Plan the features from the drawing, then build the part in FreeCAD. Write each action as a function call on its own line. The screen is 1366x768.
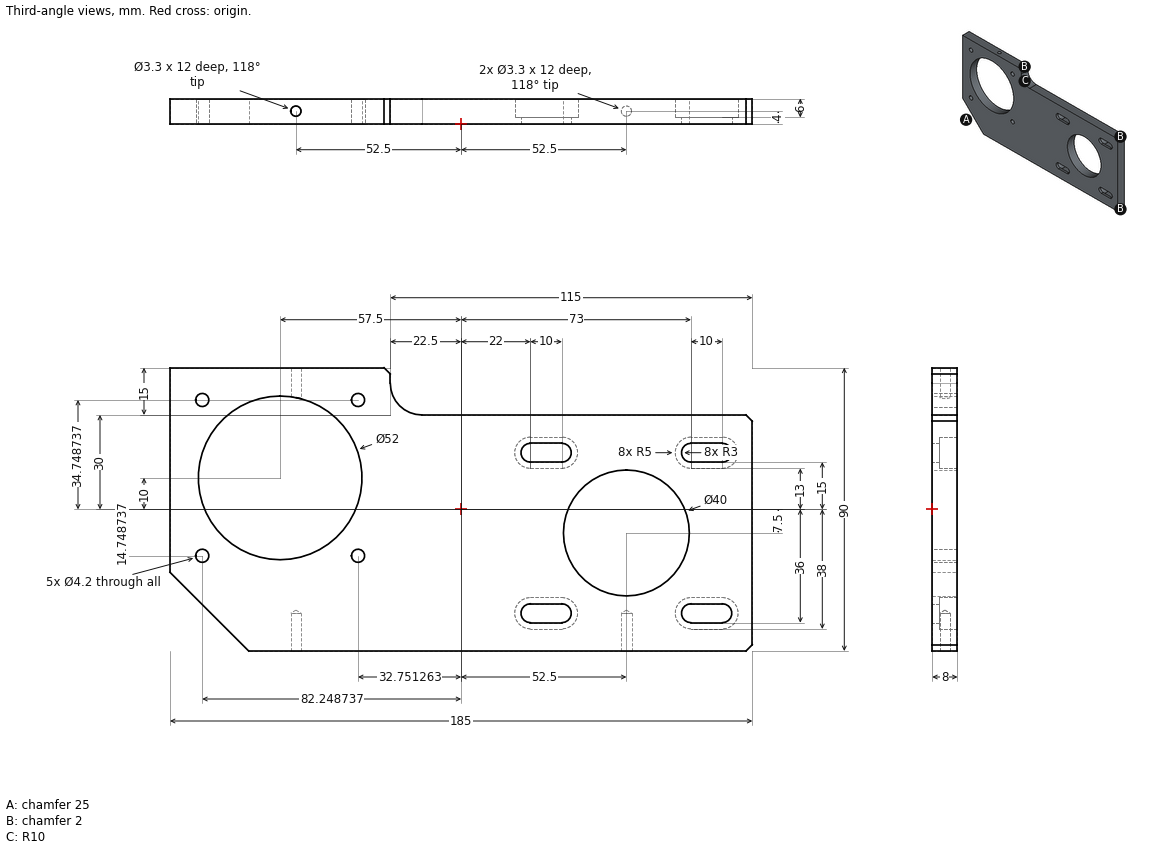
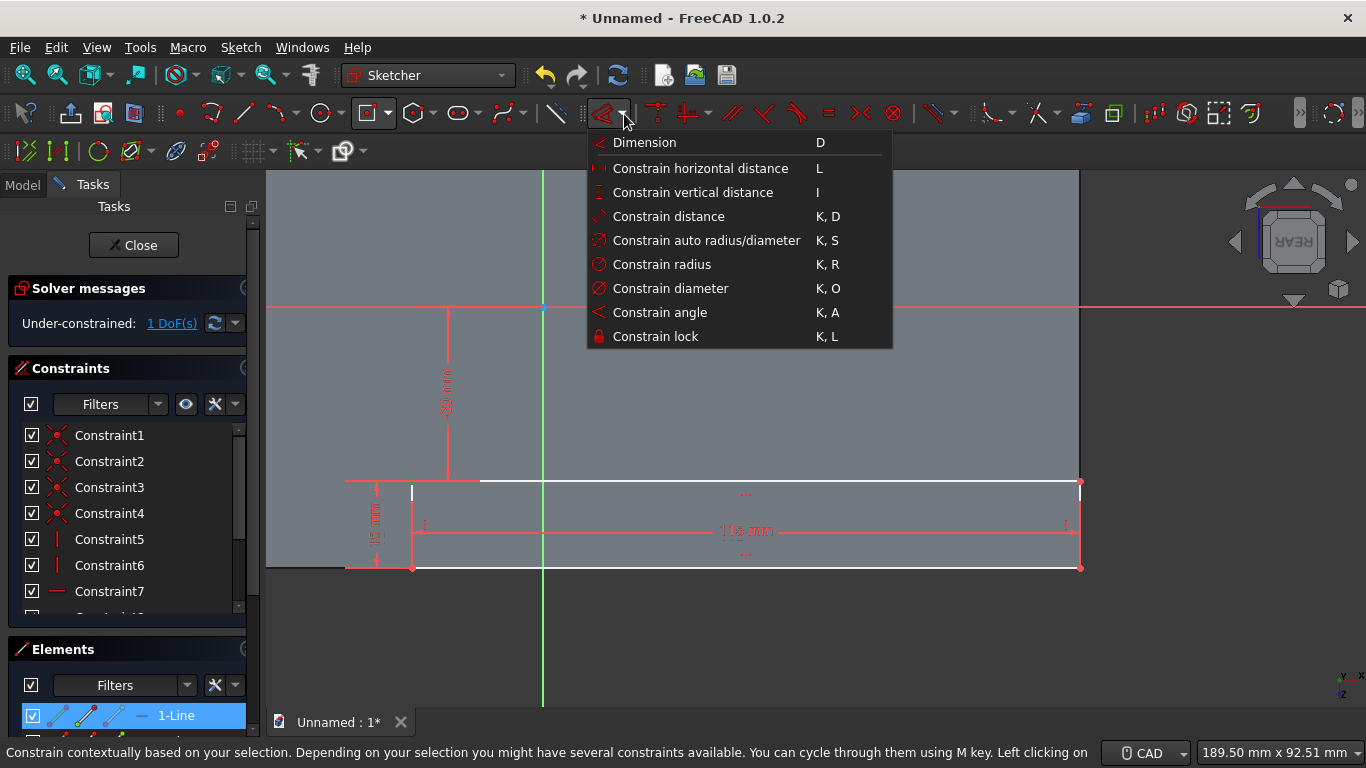
click(740, 168)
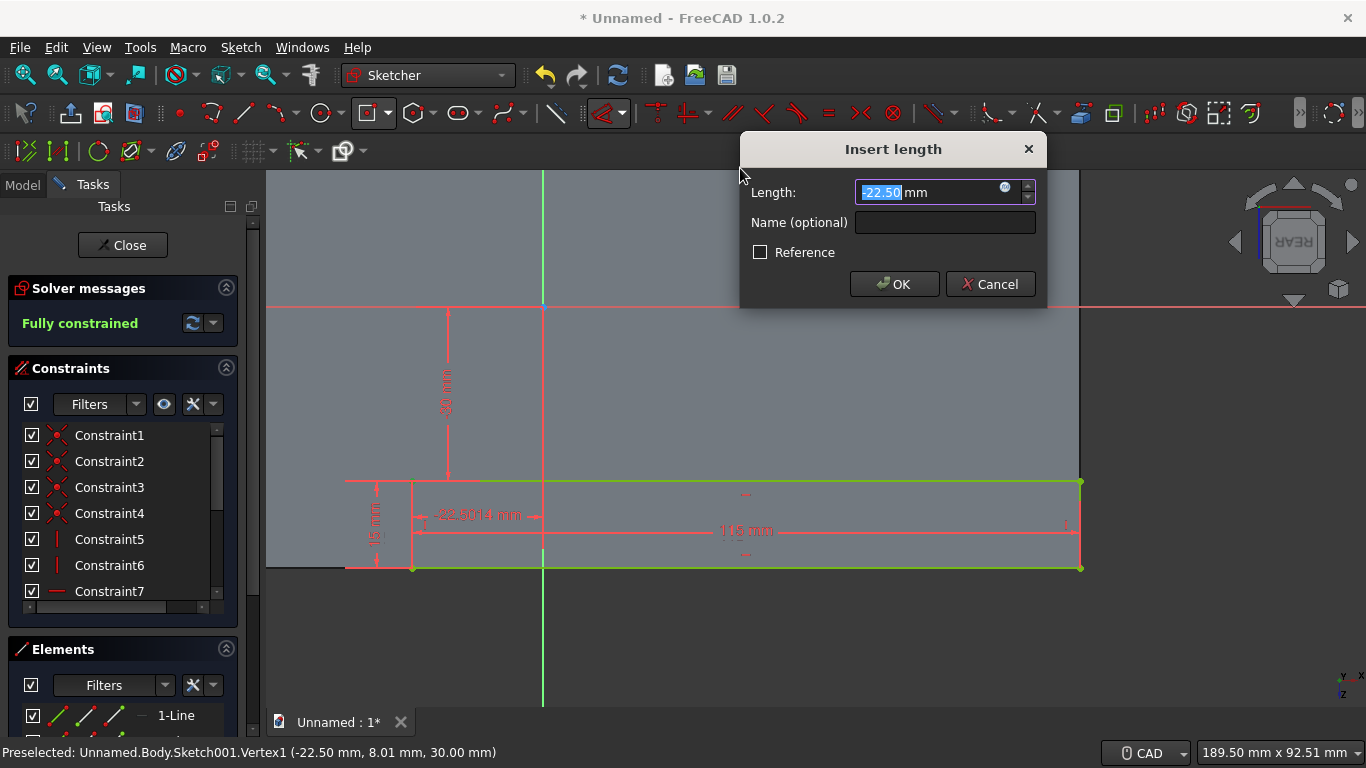
text(-22.5)
key(Return)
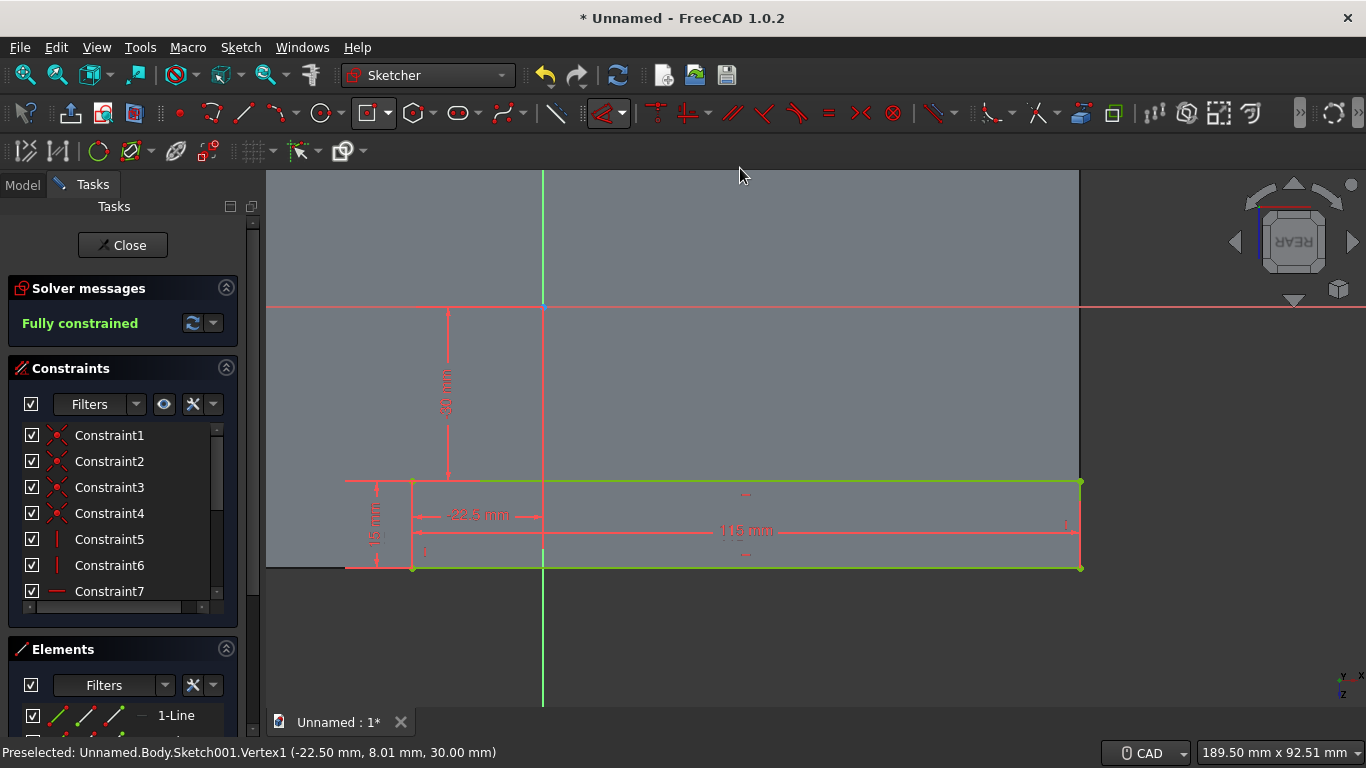
click(123, 245)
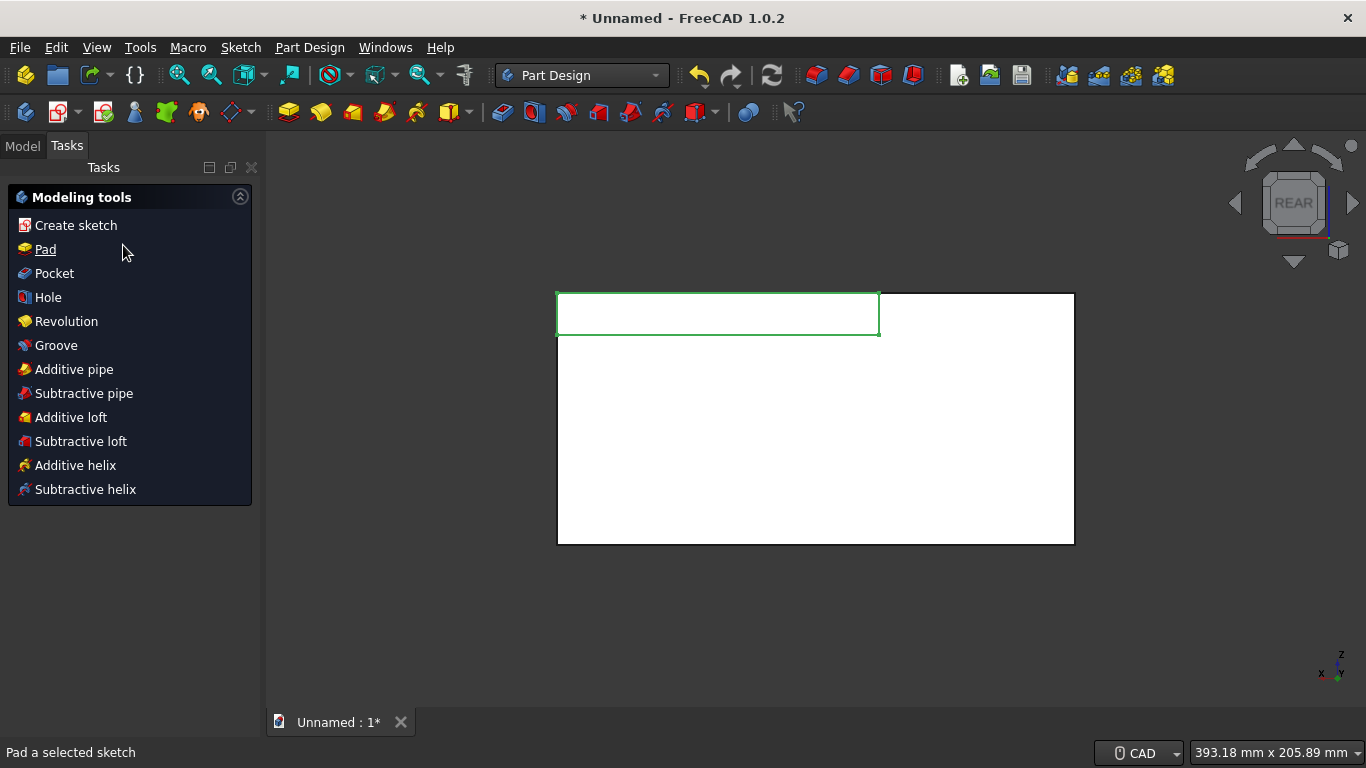
click(504, 112)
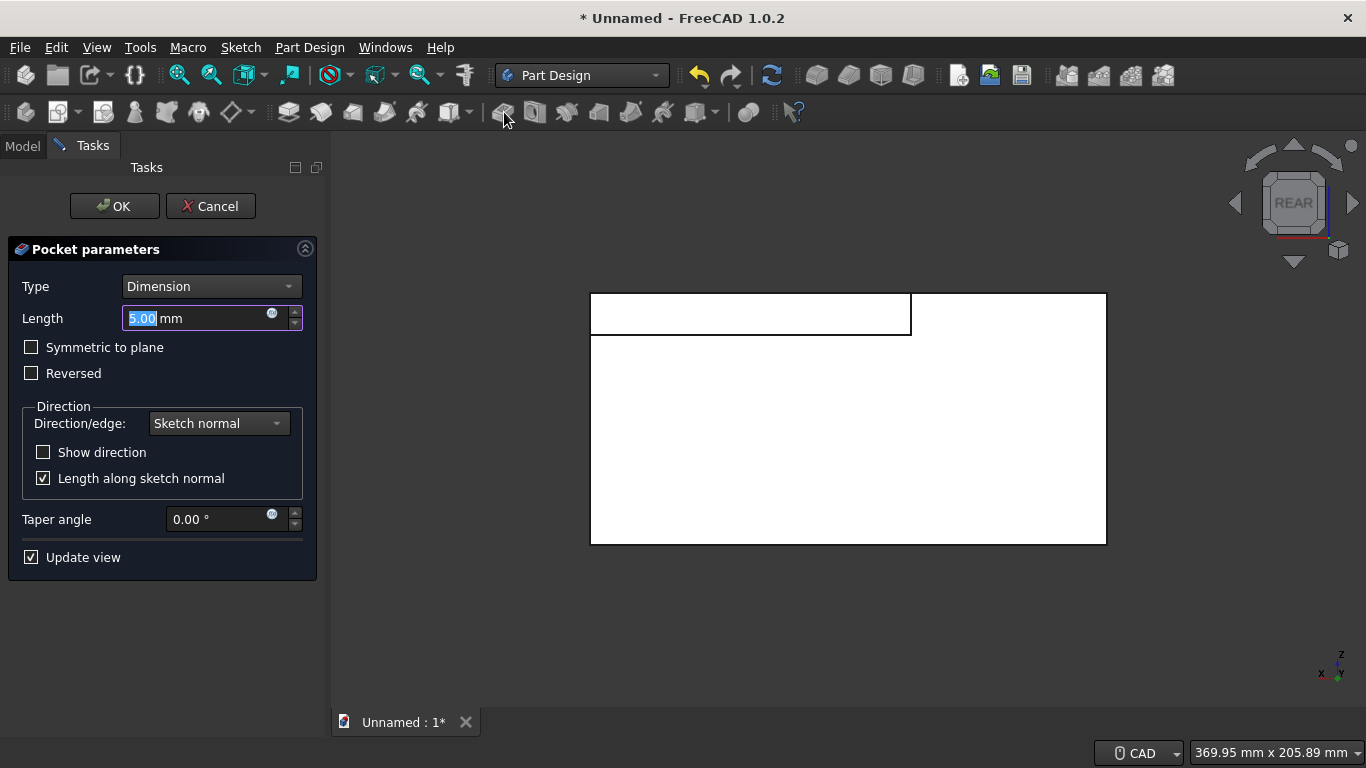
click(212, 286)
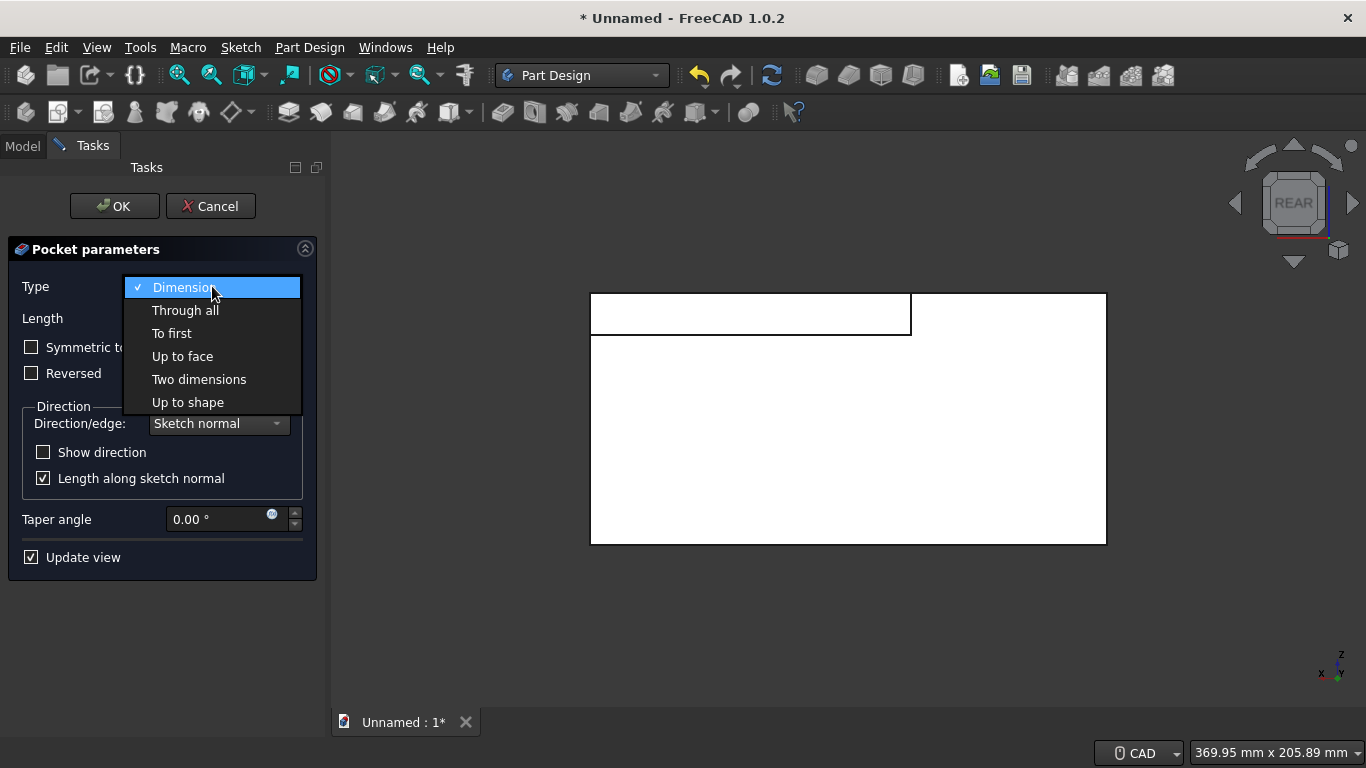
click(212, 310)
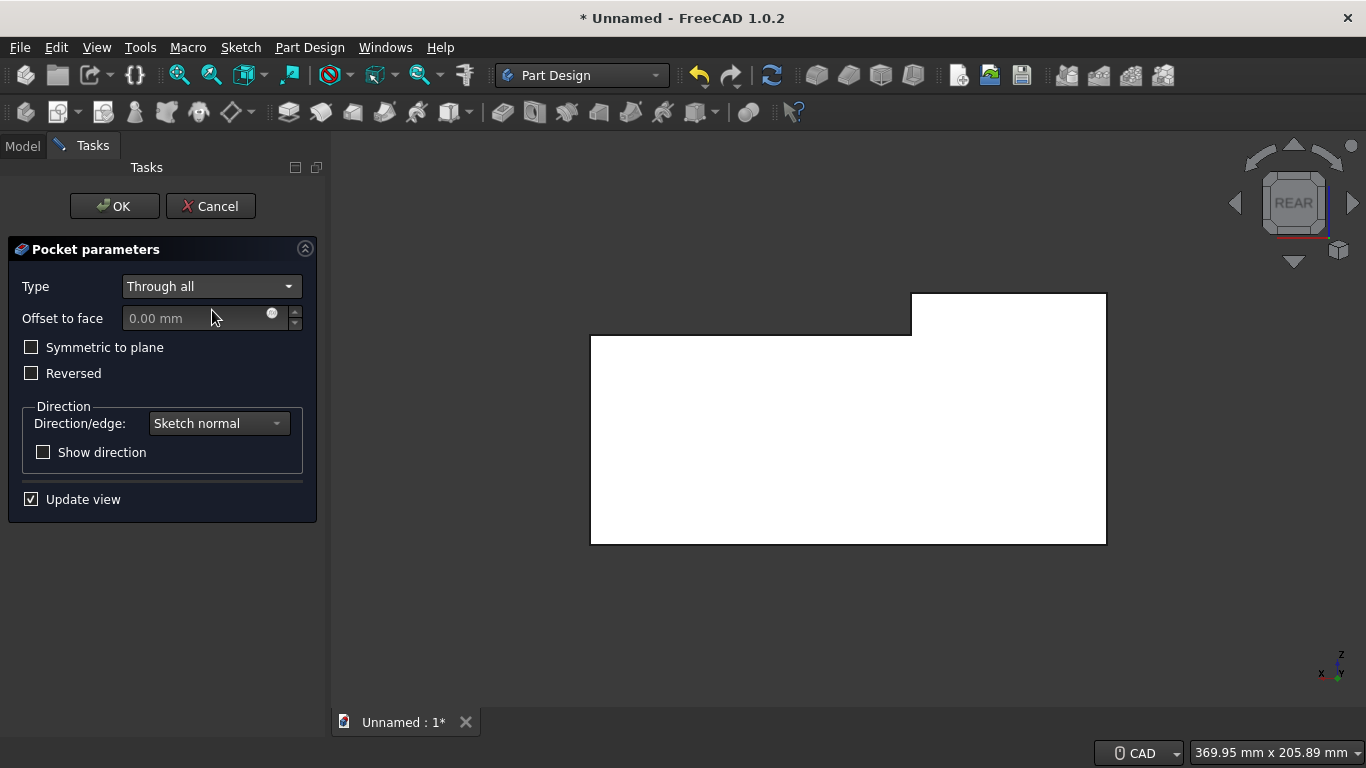
click(115, 206)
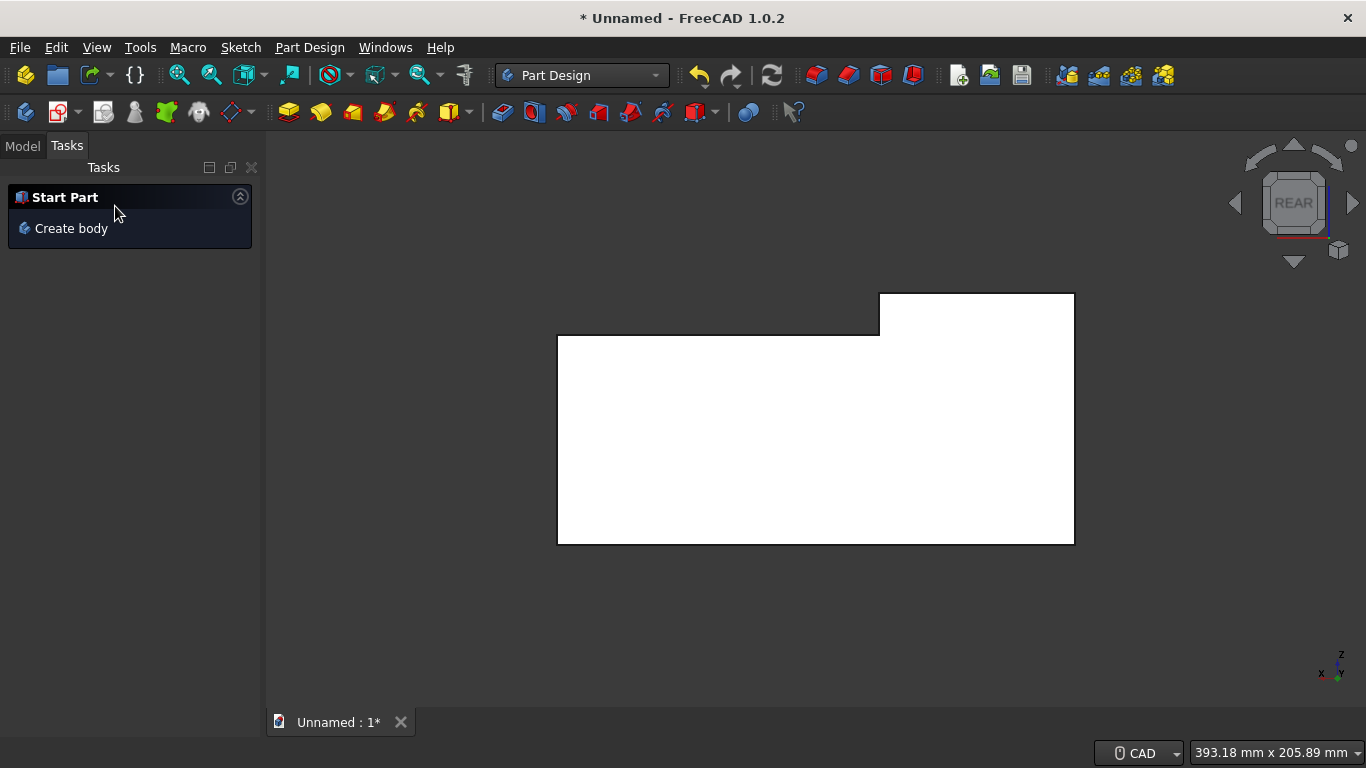
click(964, 418)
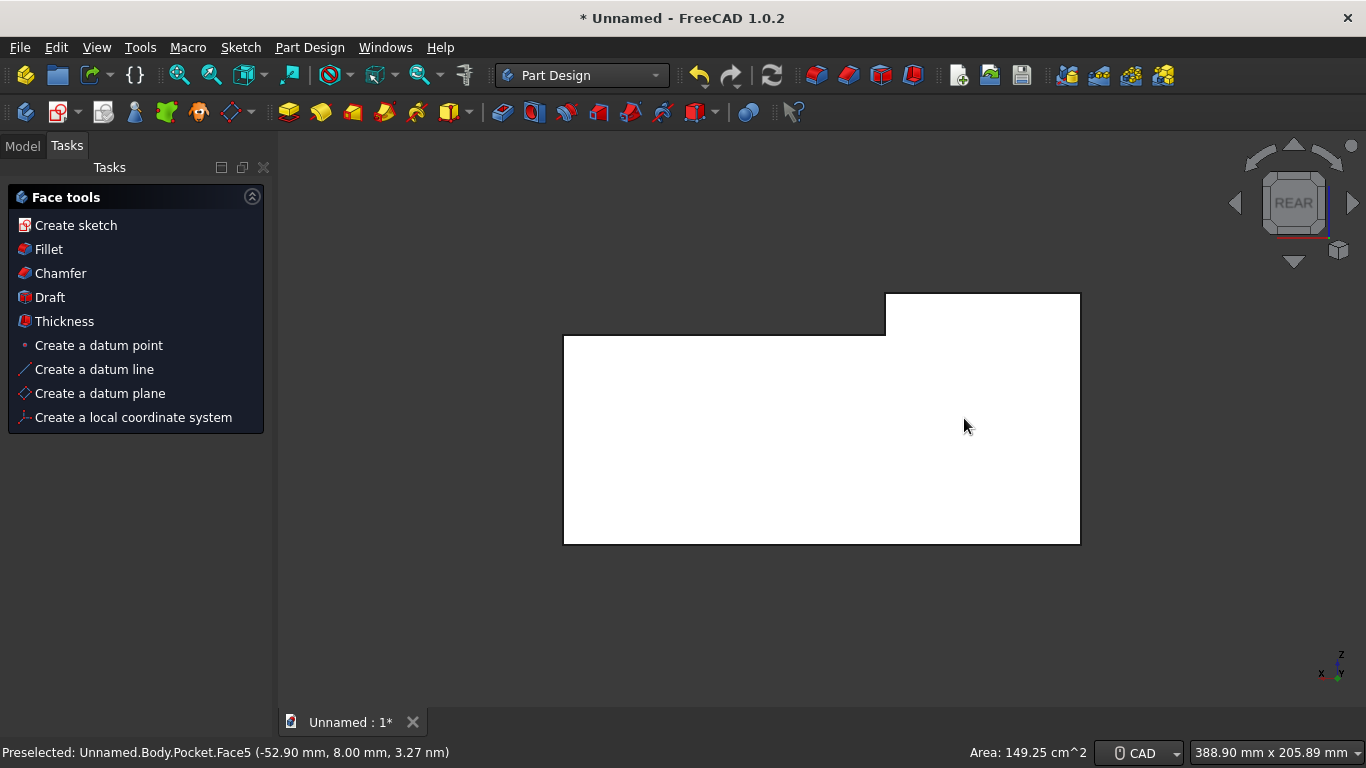
click(58, 112)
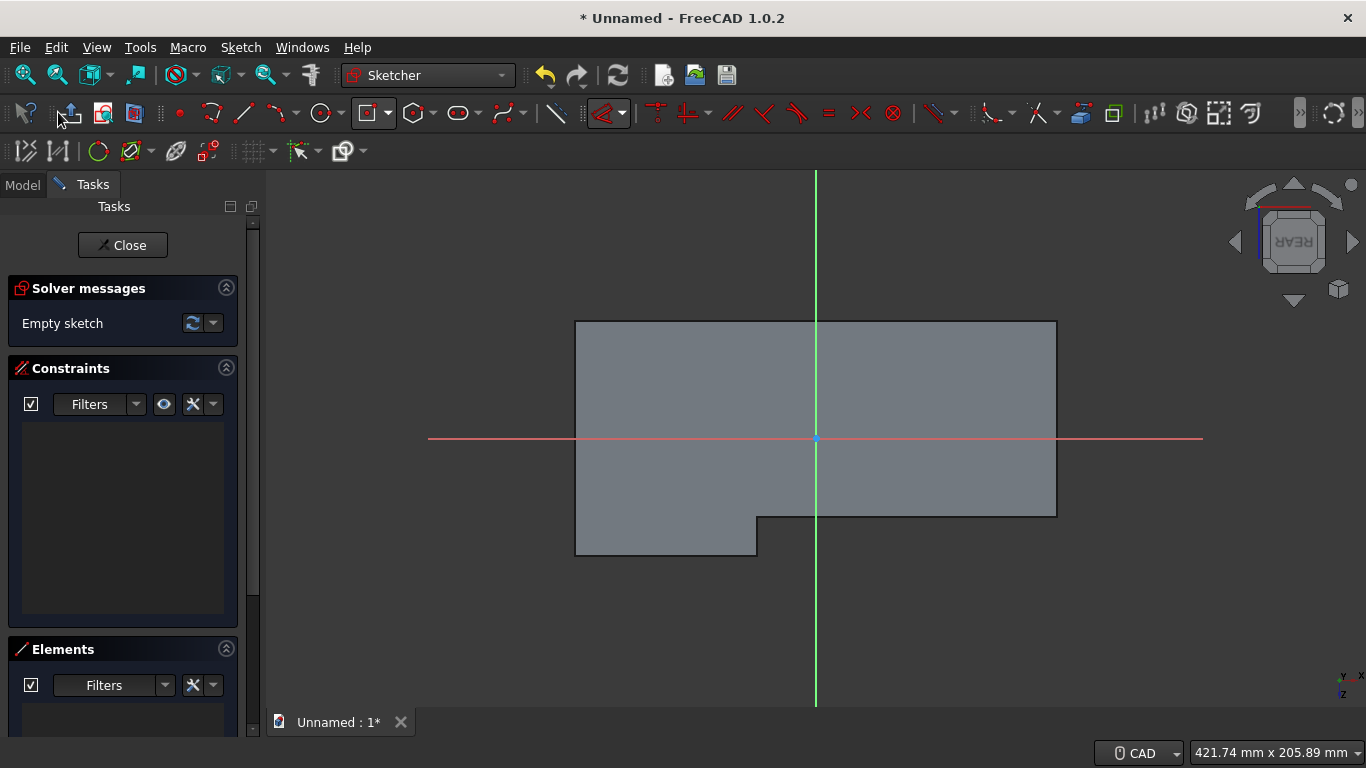
scroll(684, 480, up, 5)